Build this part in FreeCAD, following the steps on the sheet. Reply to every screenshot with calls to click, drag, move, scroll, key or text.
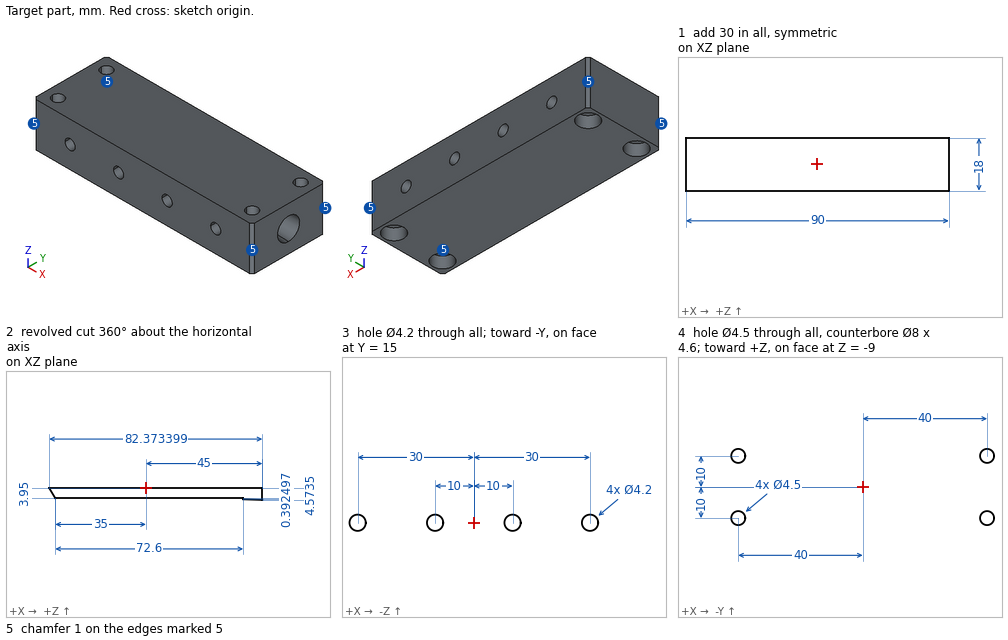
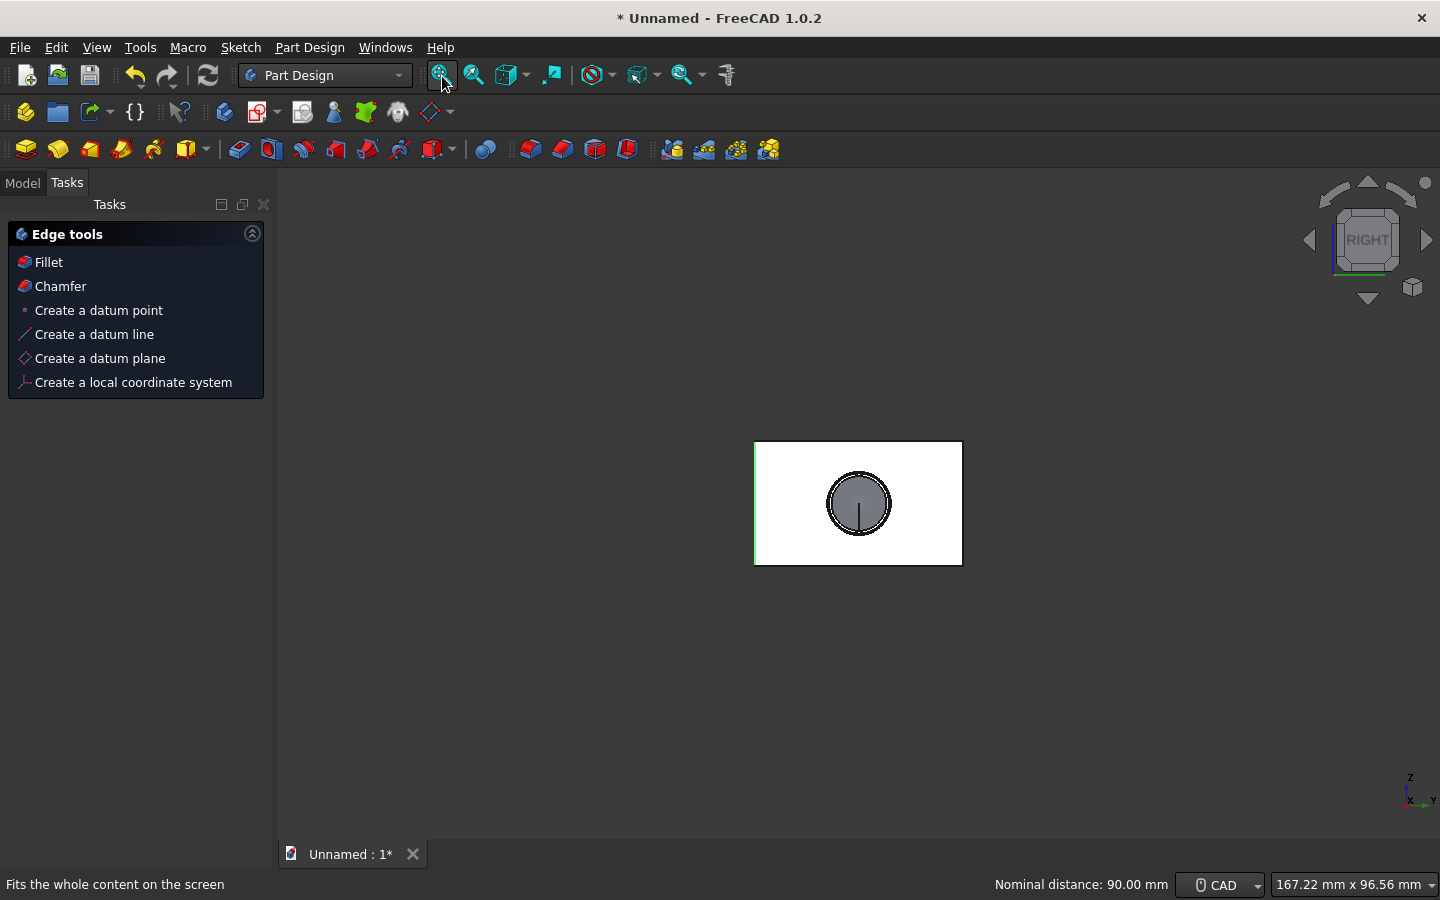
click(963, 502, ctrl)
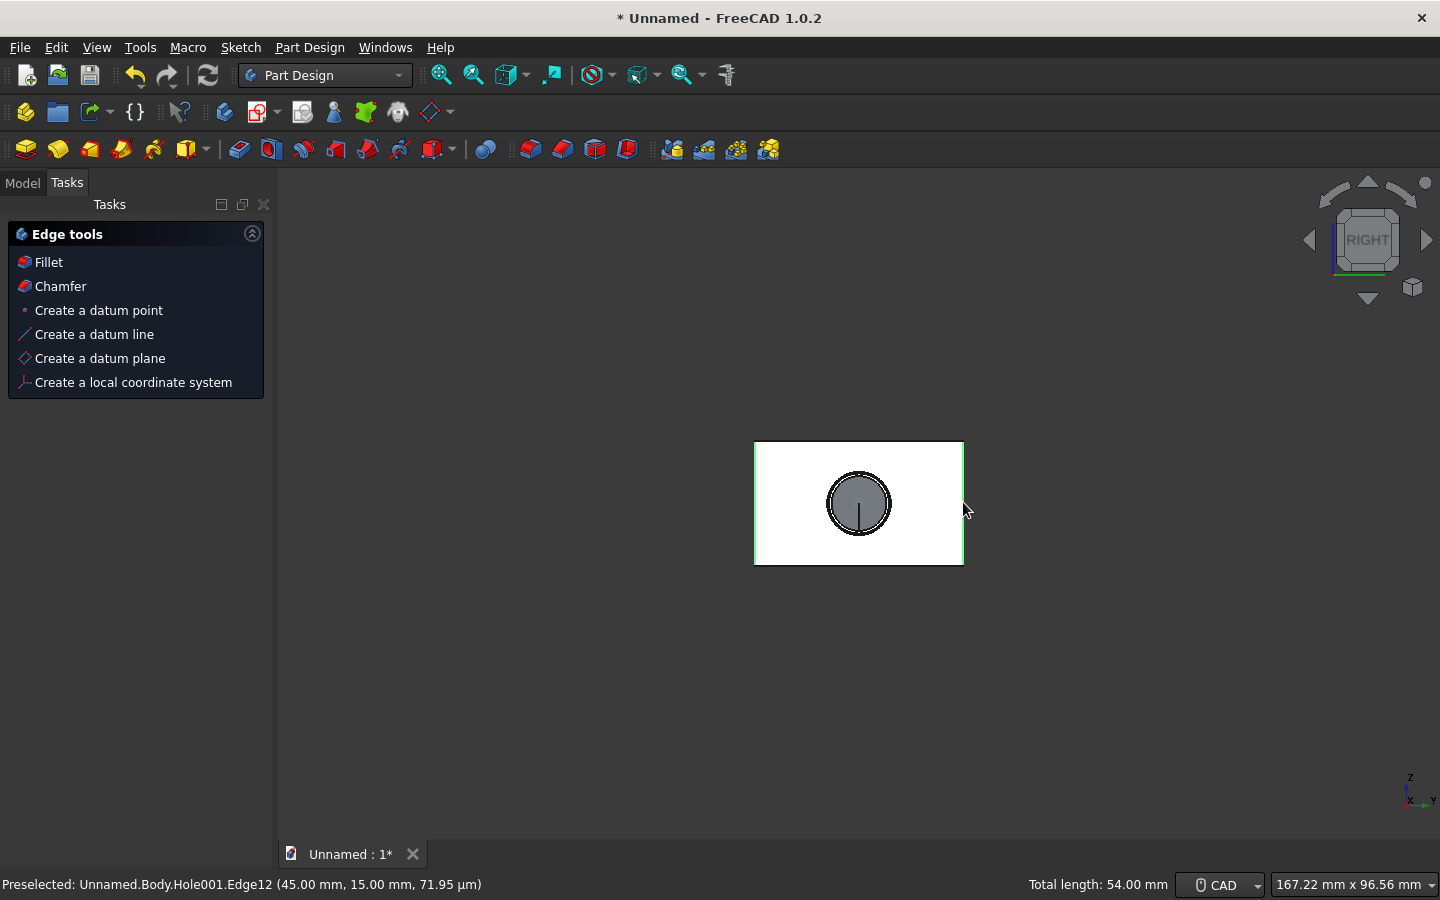
key(5)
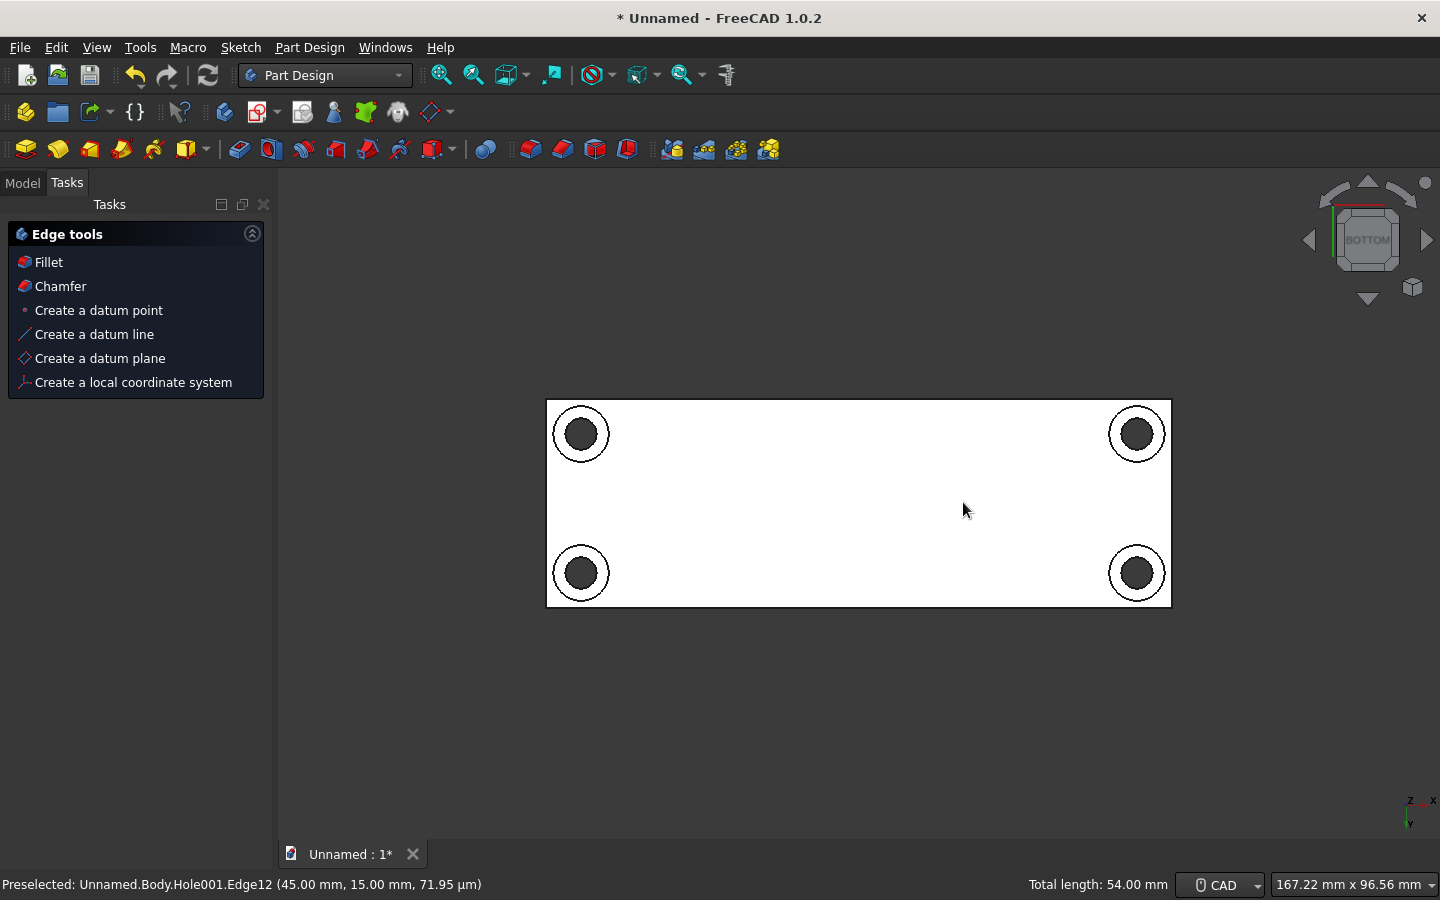
key(4)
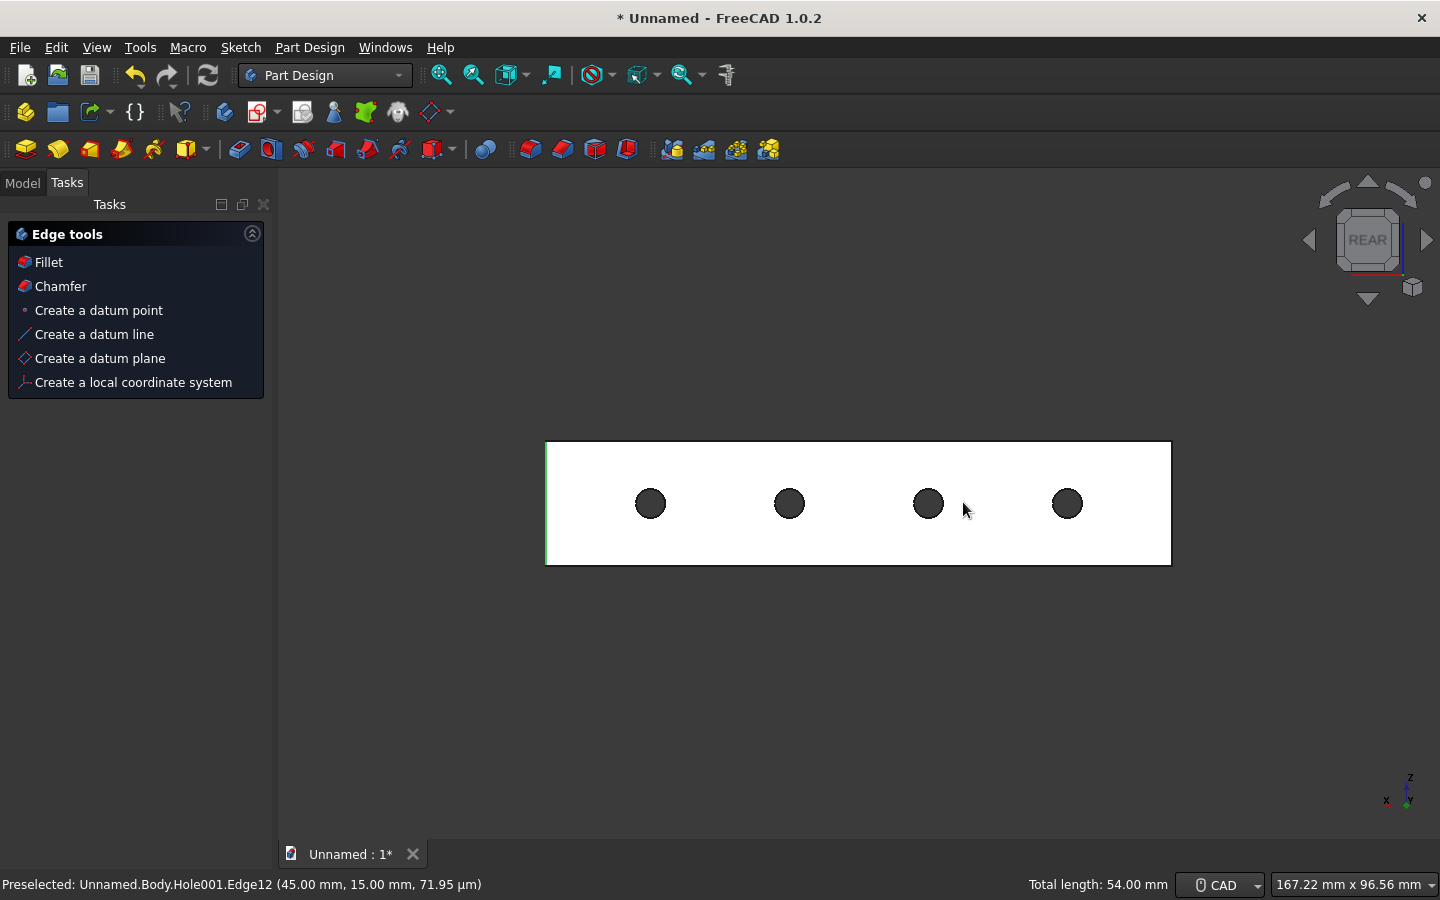
click(1172, 502, ctrl)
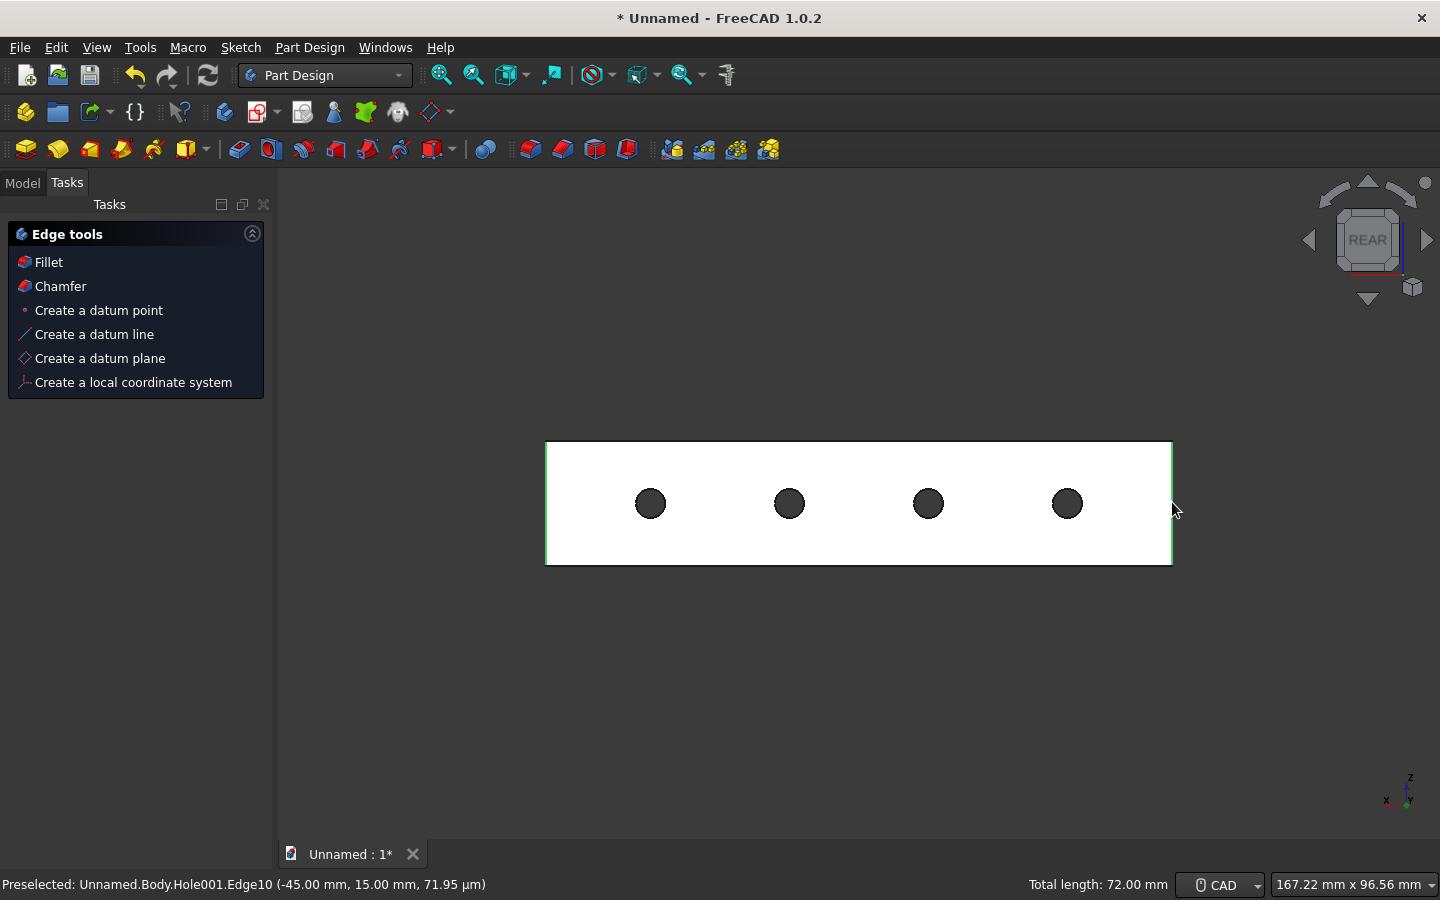
click(564, 150)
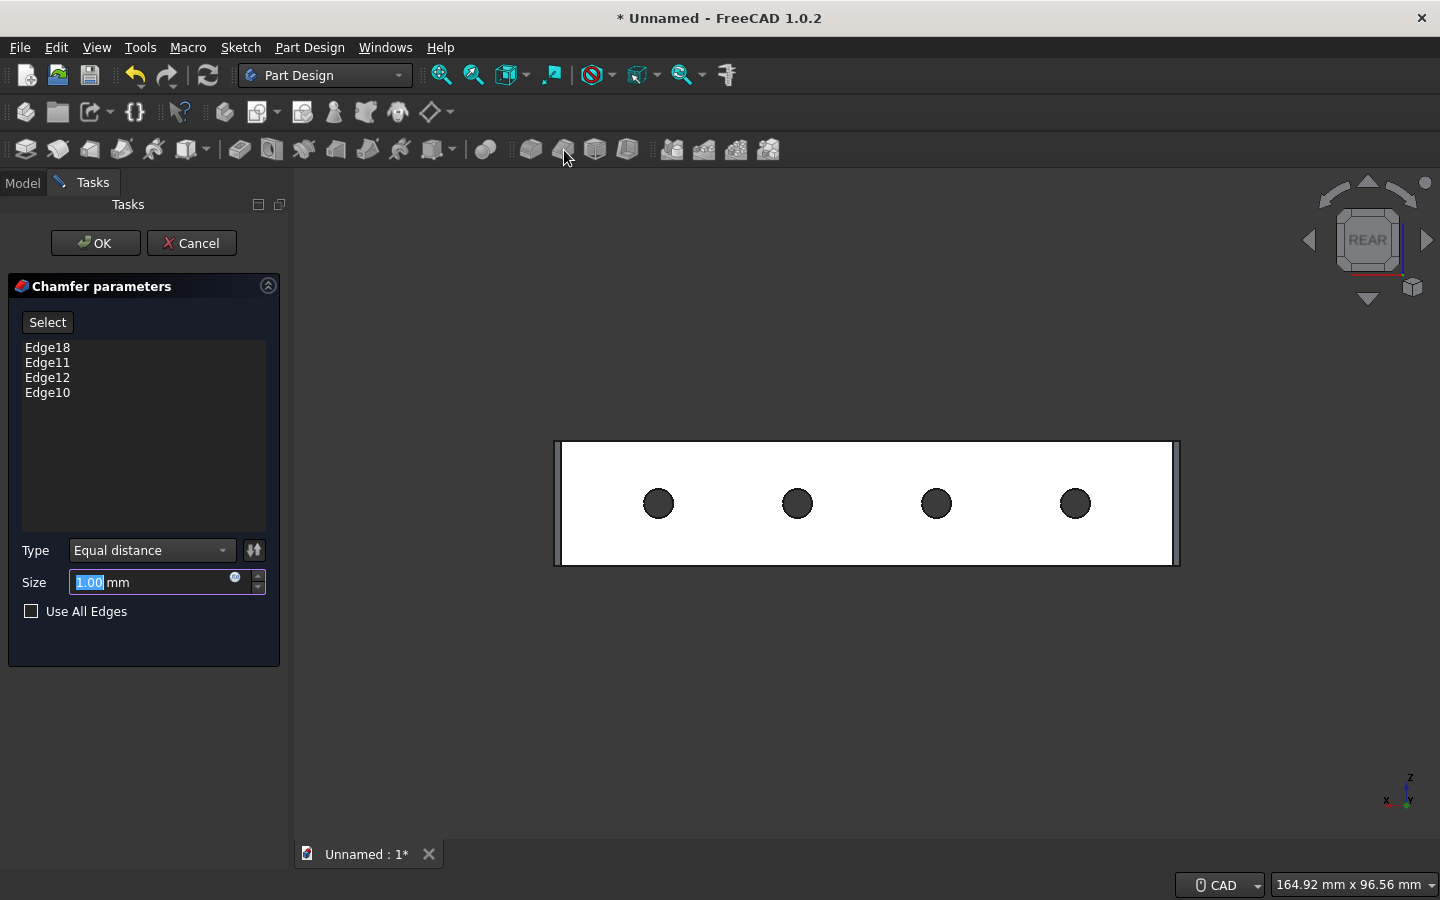
text(1)
key(Tab)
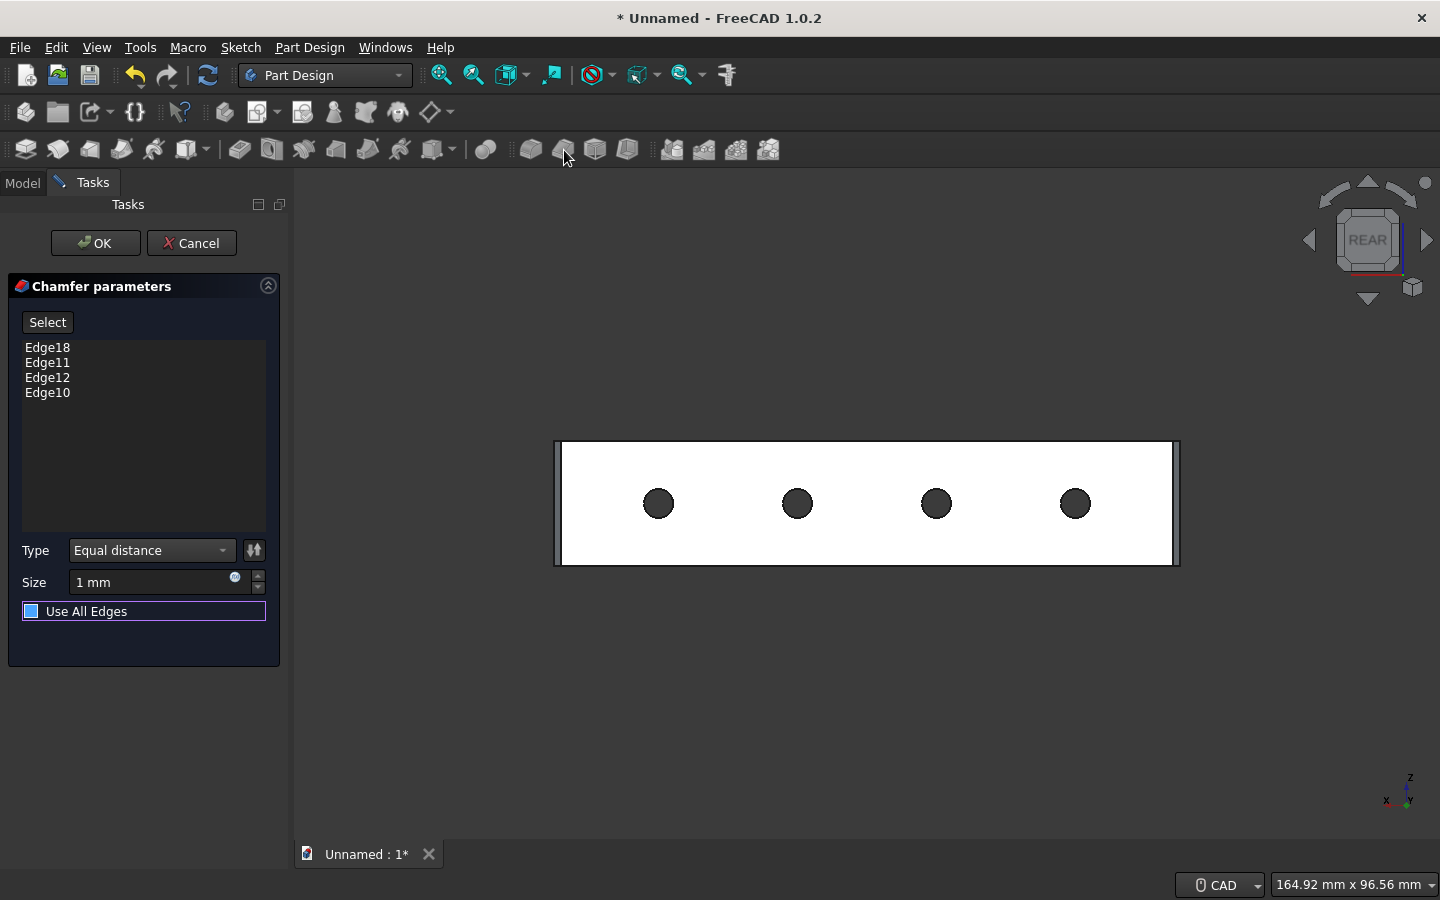
click(96, 243)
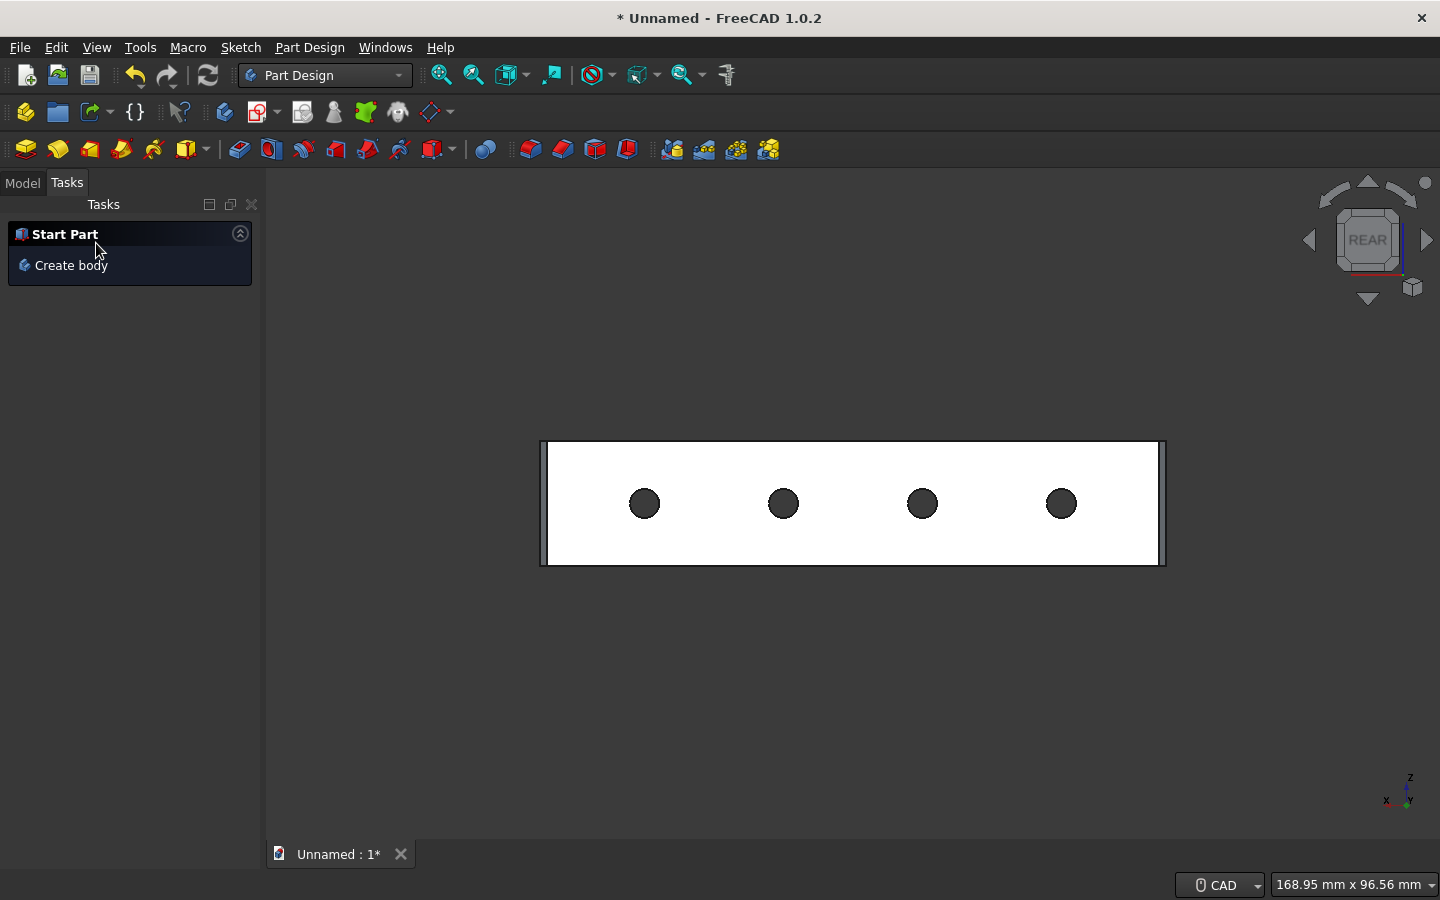
key(0)